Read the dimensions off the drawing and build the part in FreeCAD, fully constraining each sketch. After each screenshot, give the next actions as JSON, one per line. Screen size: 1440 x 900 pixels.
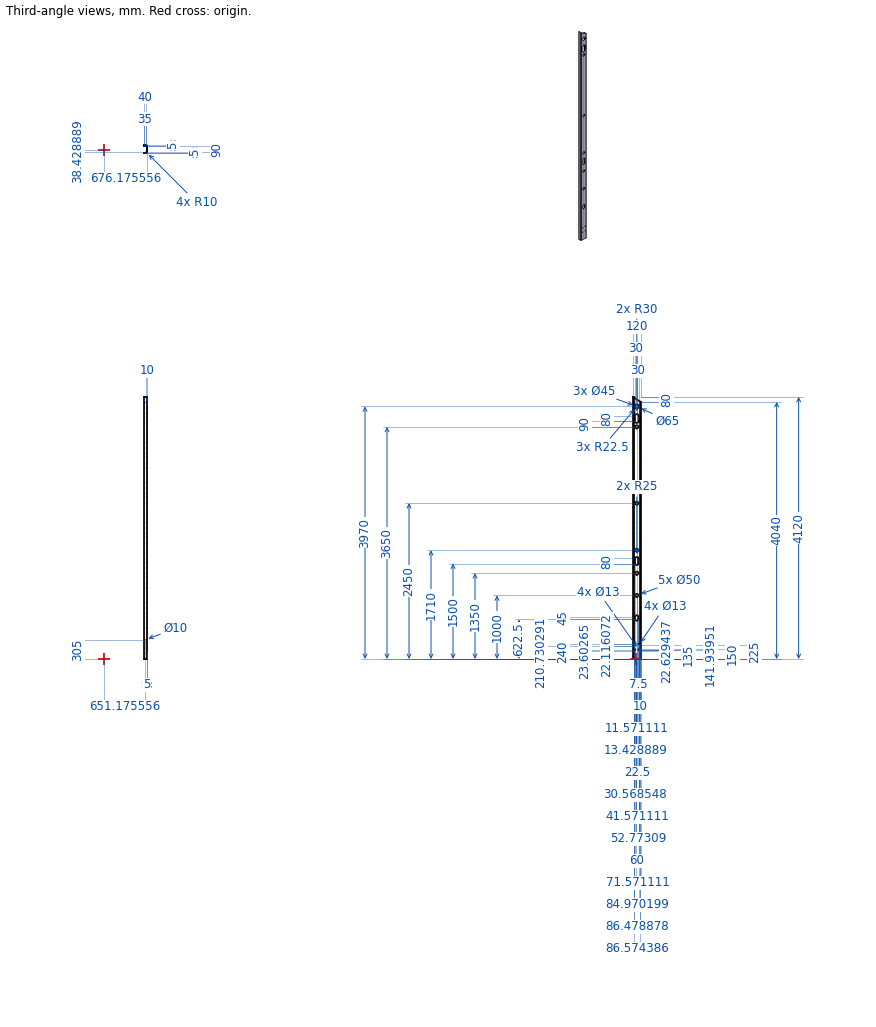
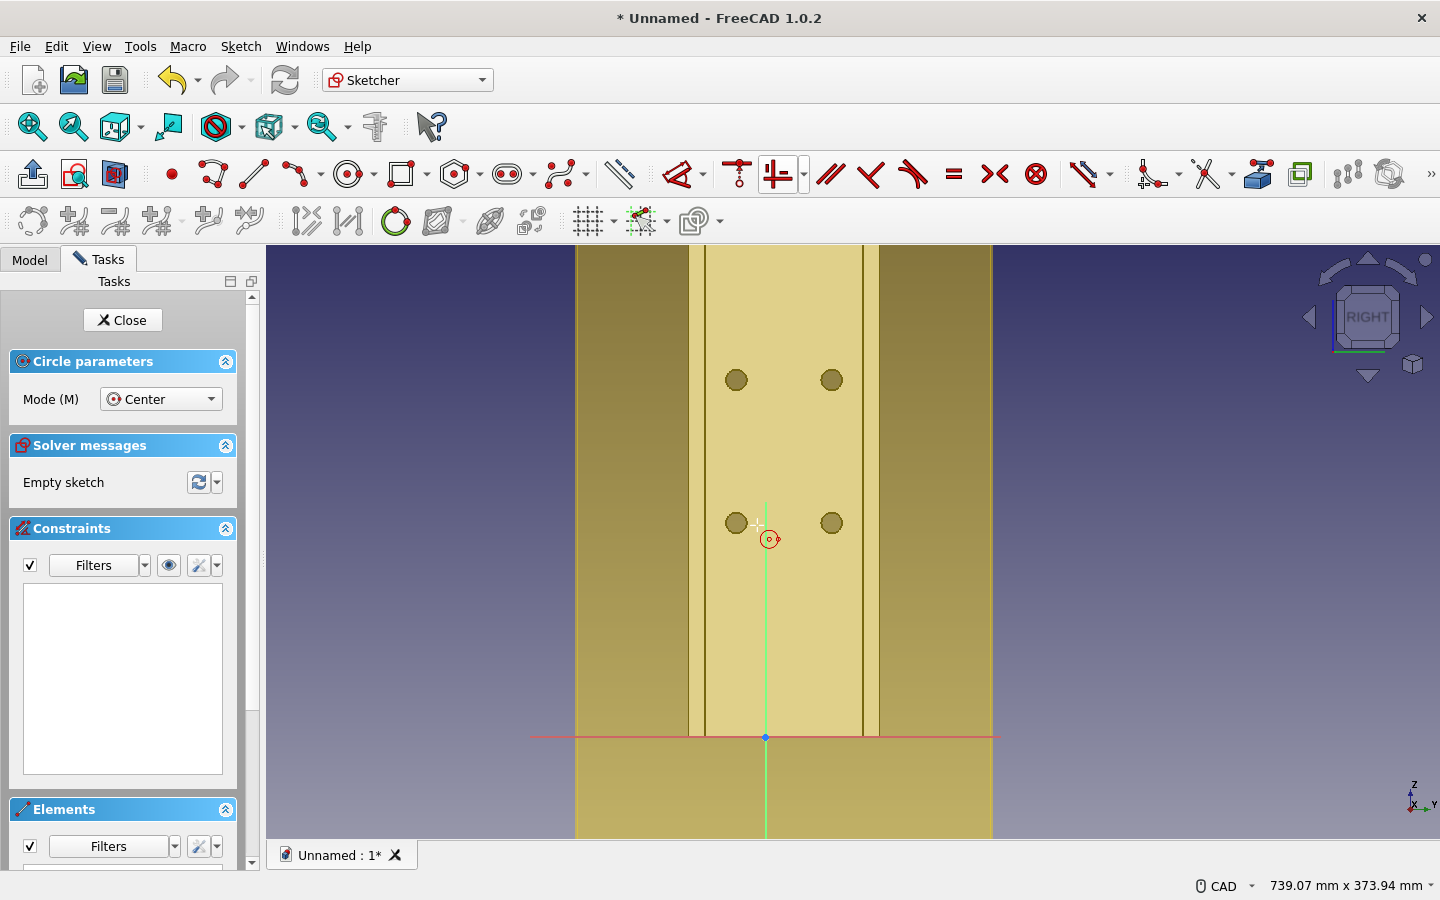
{"action": "scroll", "coordinate": [832, 499], "scroll_direction": "up", "scroll_amount": 4}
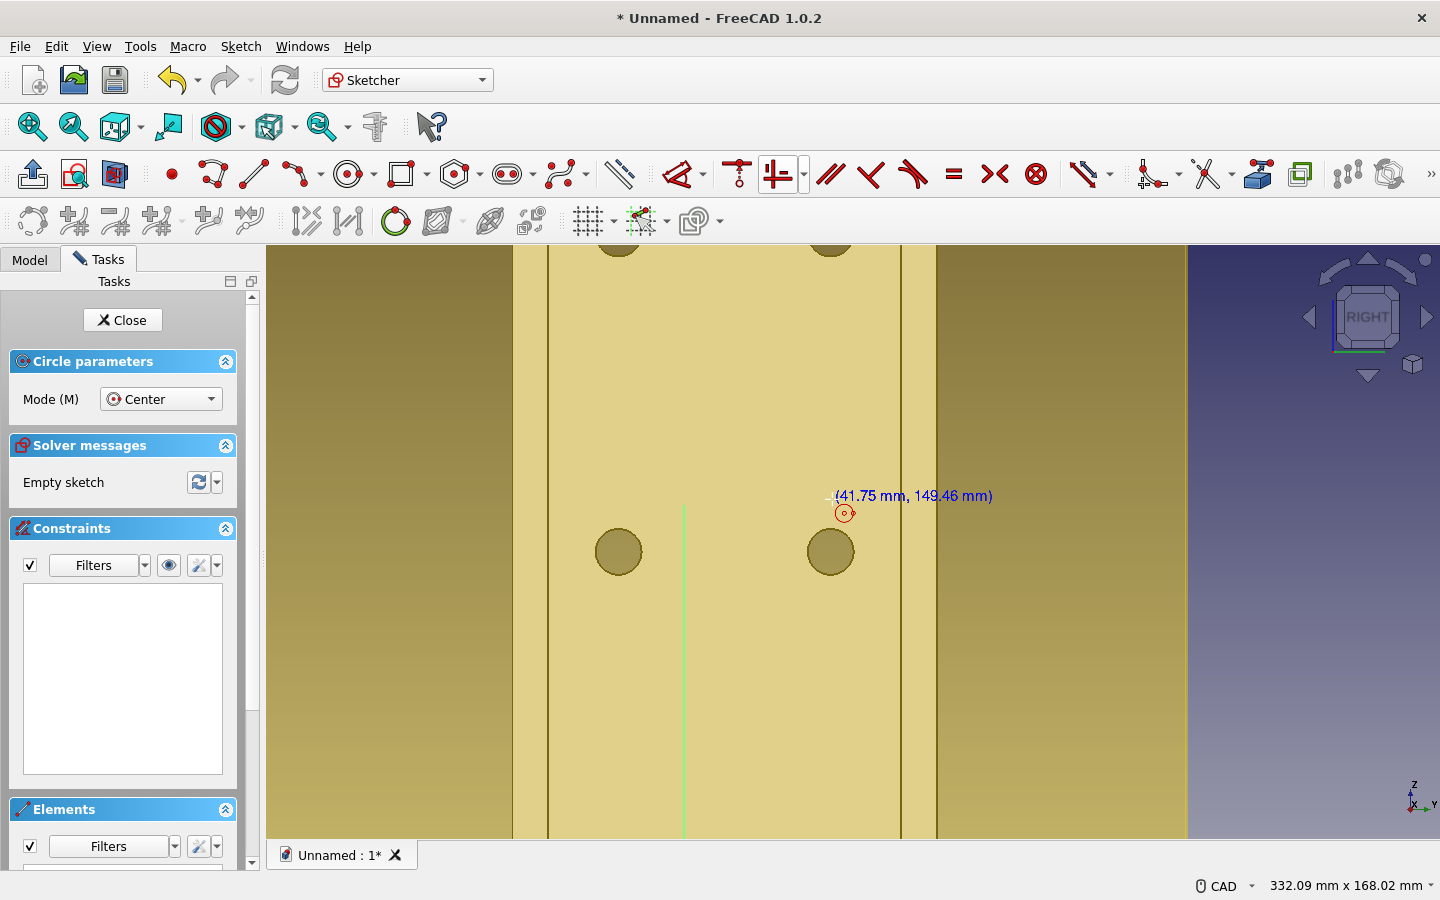
{"action": "left_click", "coordinate": [831, 499]}
{"action": "mouse_move", "coordinate": [847, 483]}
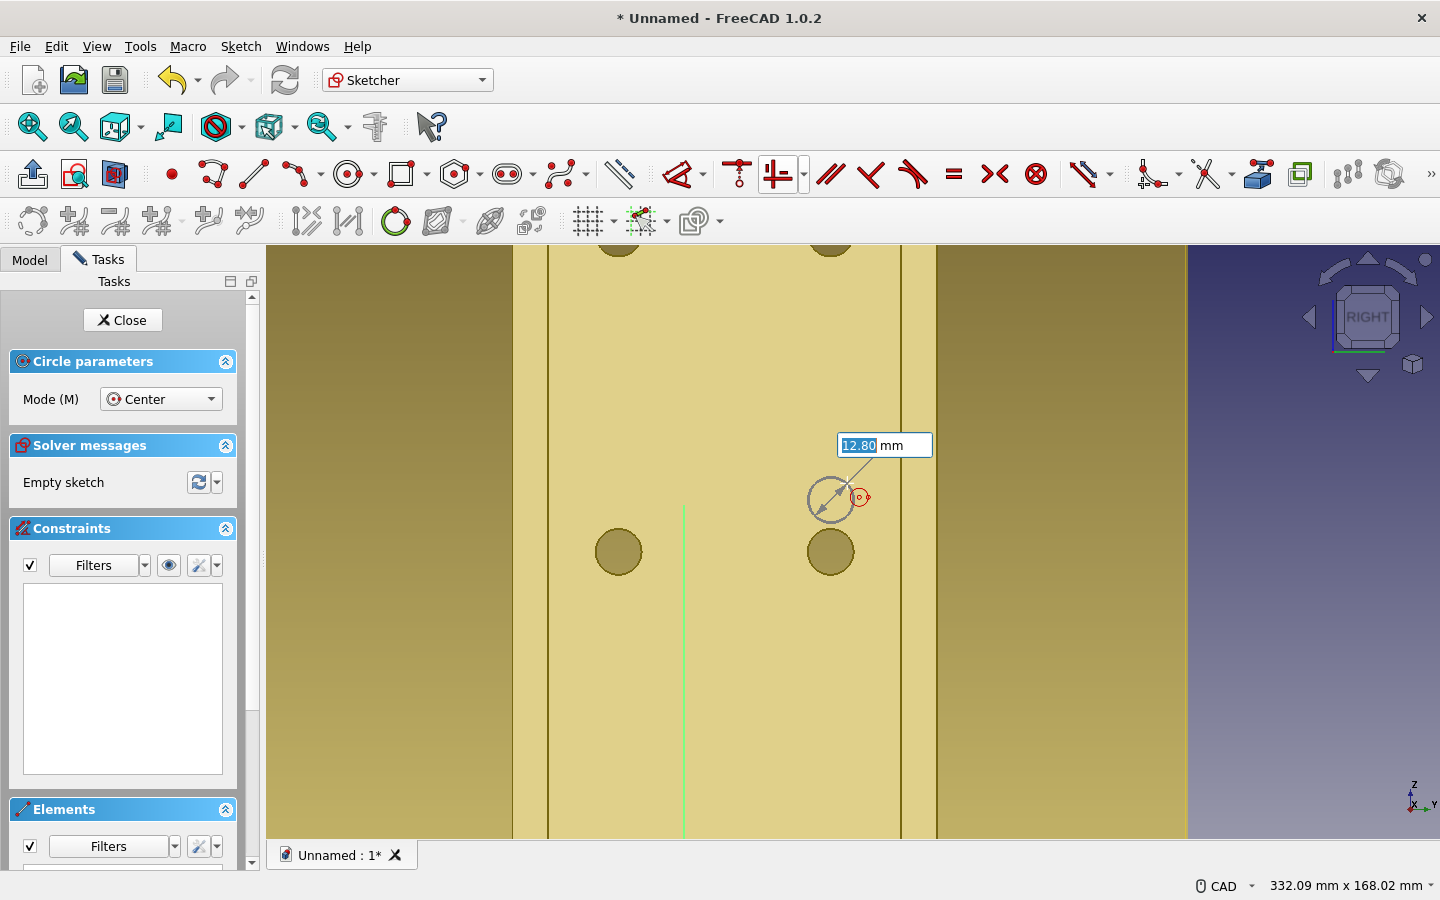
{"action": "type", "text": "13"}
{"action": "key", "text": "Return"}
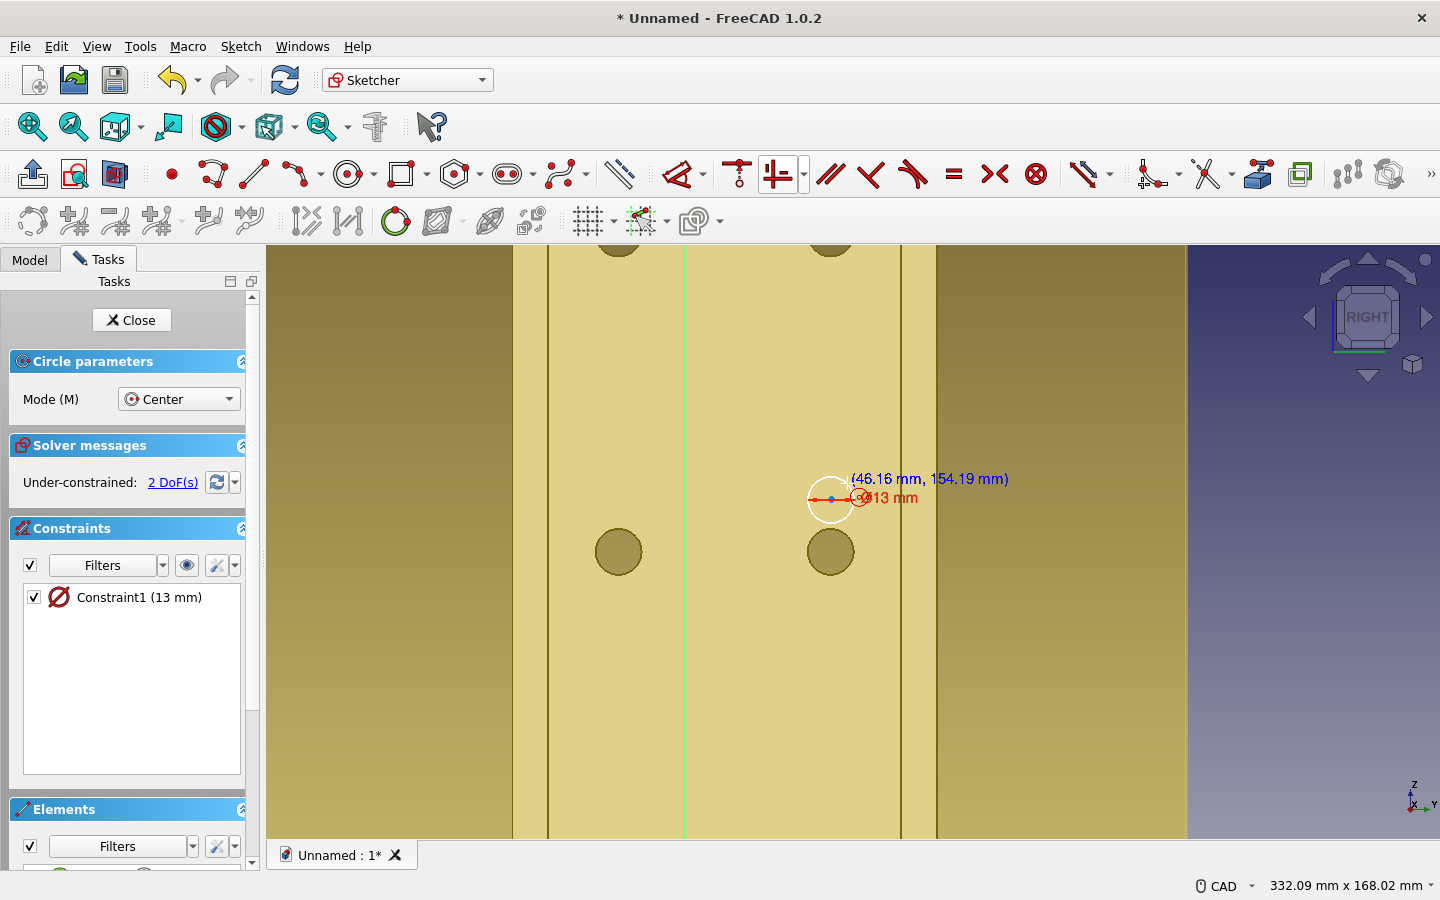
{"action": "left_click", "coordinate": [619, 499]}
{"action": "mouse_move", "coordinate": [635, 483]}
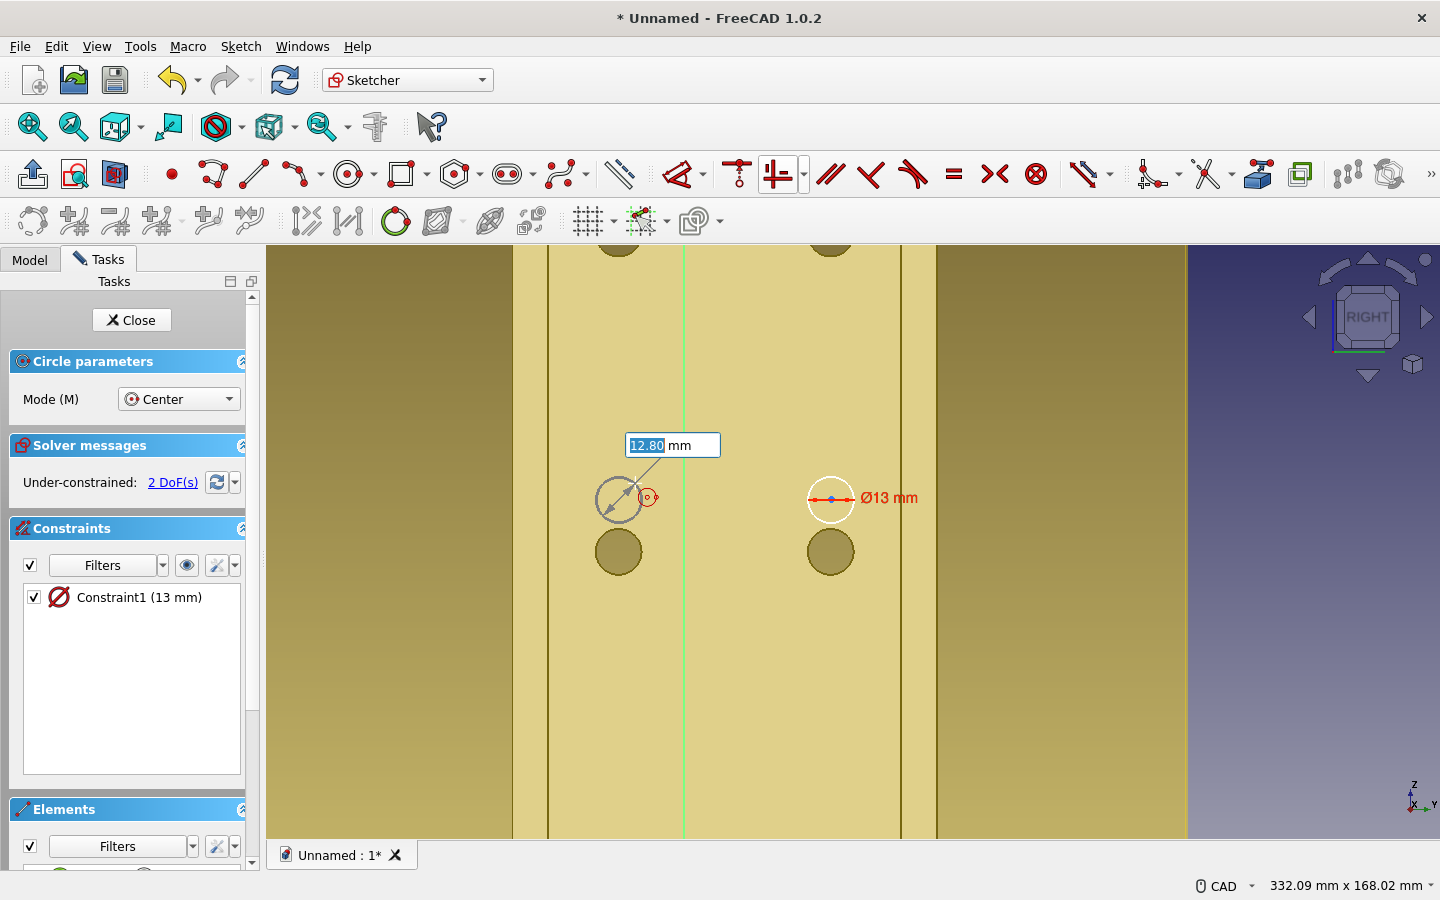
{"action": "type", "text": "13"}
{"action": "key", "text": "Return"}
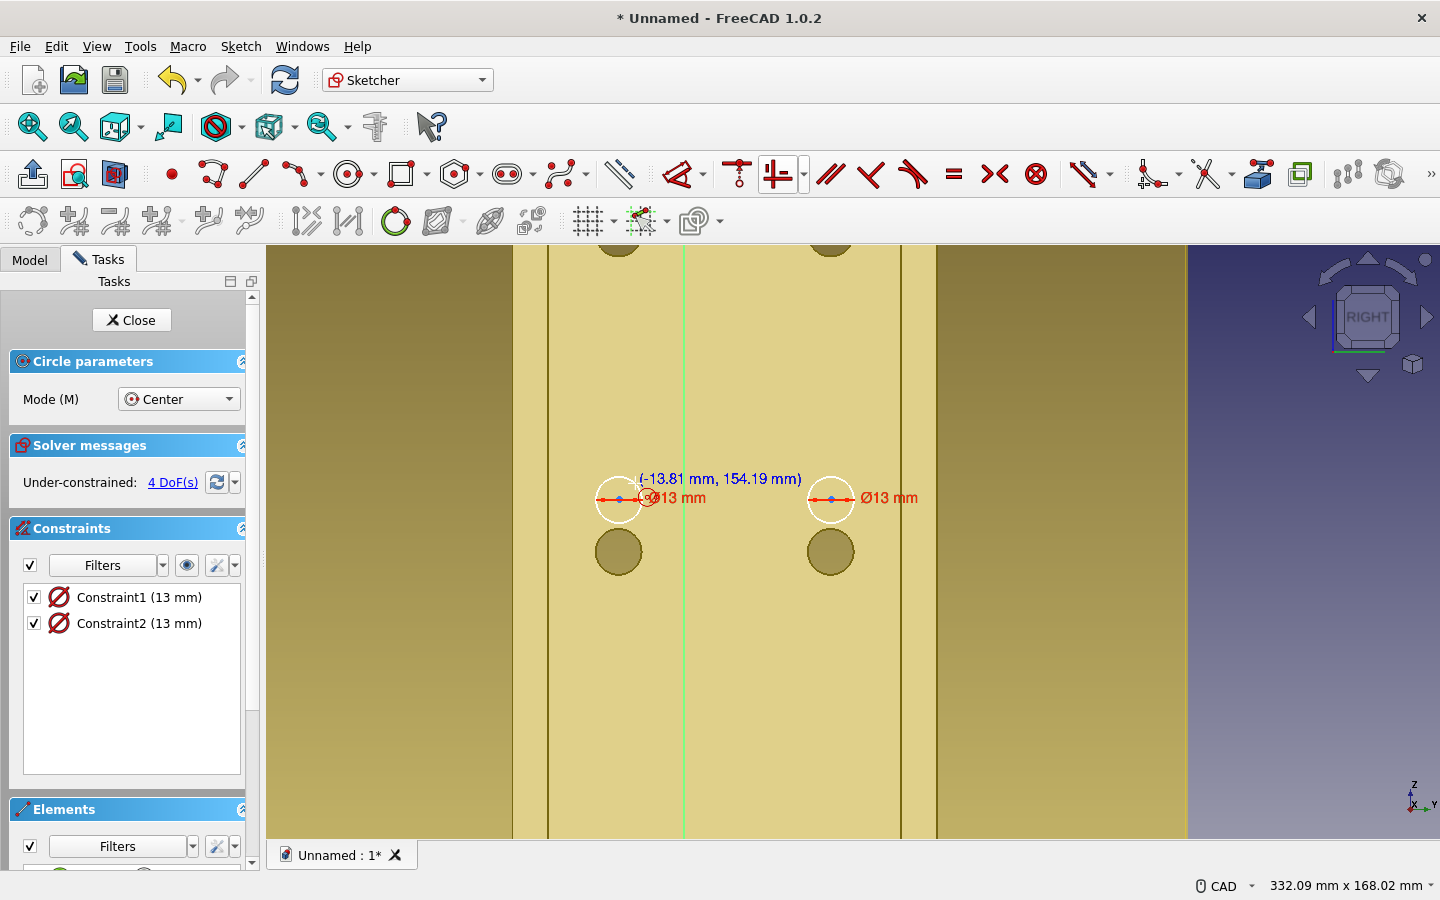
{"action": "scroll", "coordinate": [833, 500], "scroll_direction": "down", "scroll_amount": 4}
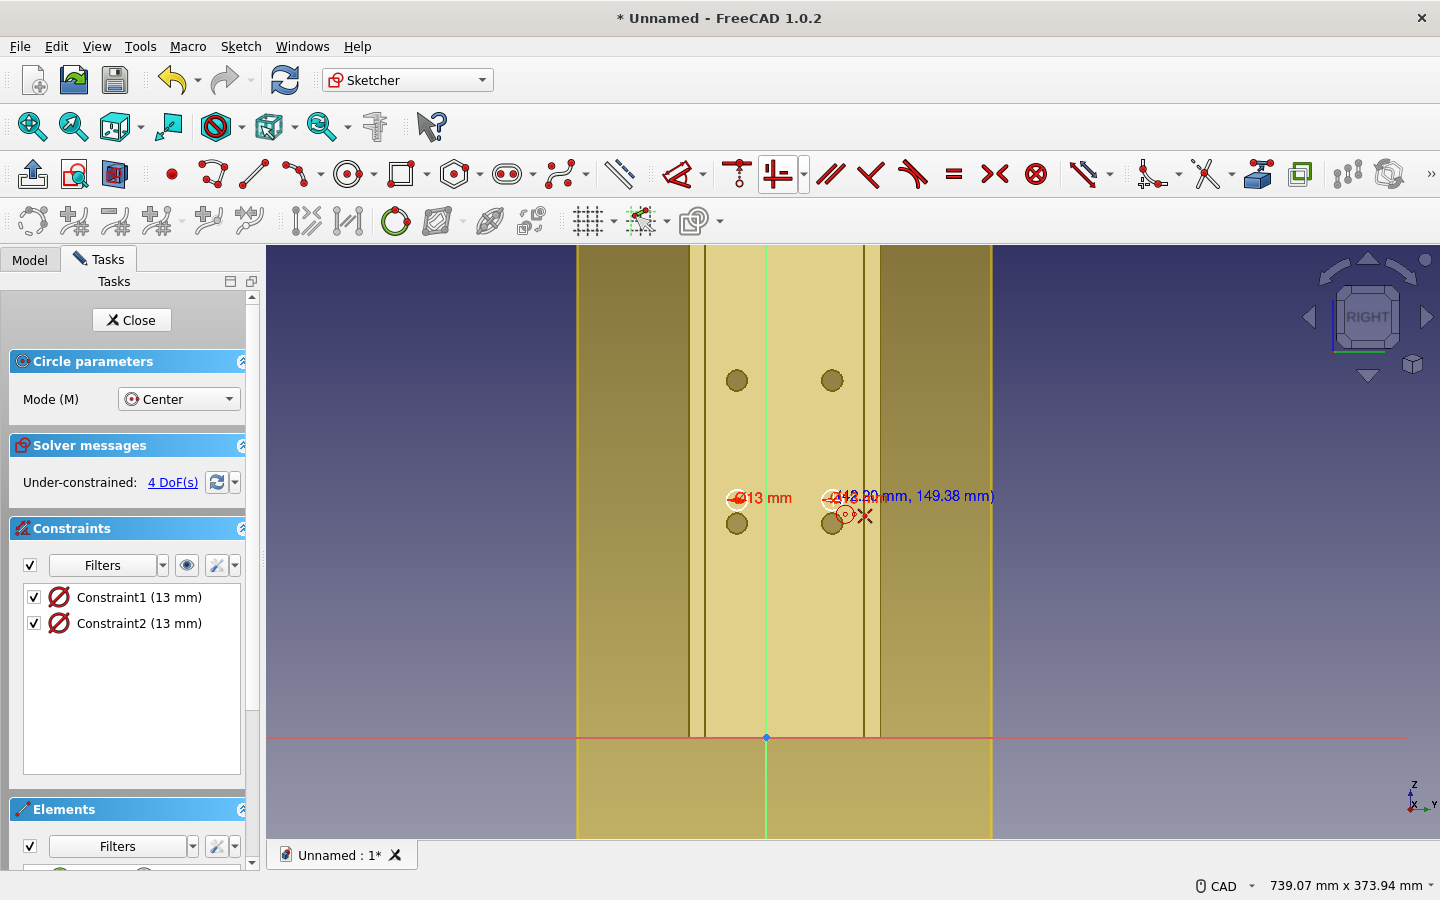
{"action": "scroll", "coordinate": [737, 357], "scroll_direction": "up", "scroll_amount": 4}